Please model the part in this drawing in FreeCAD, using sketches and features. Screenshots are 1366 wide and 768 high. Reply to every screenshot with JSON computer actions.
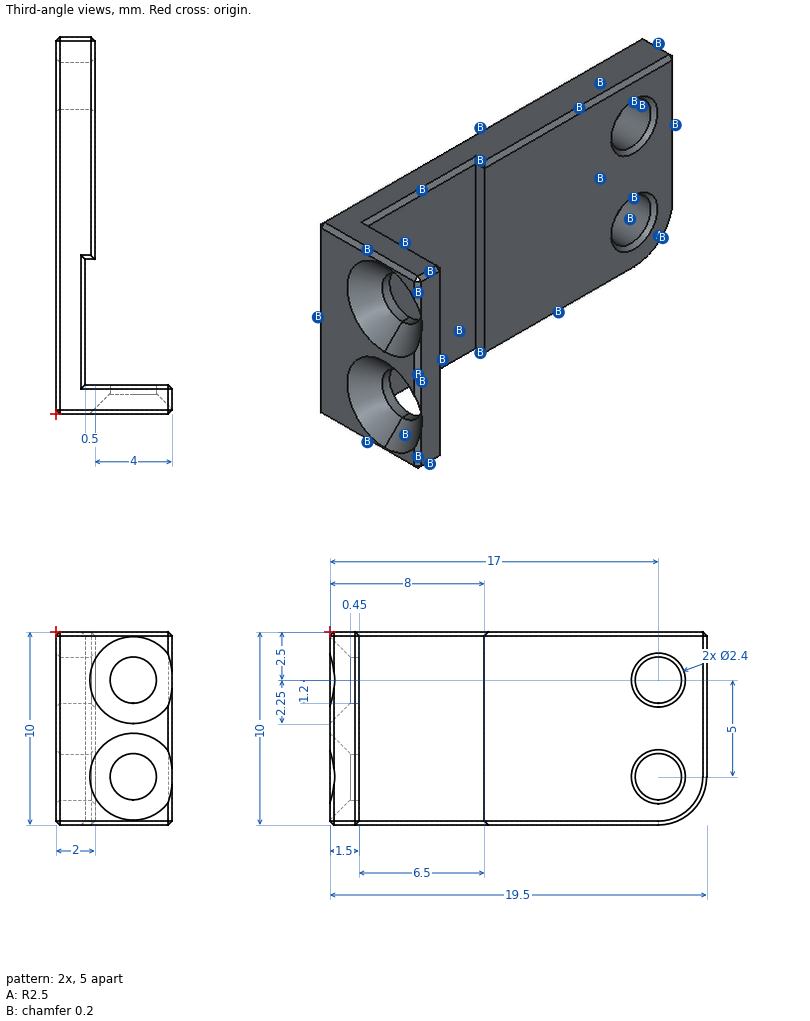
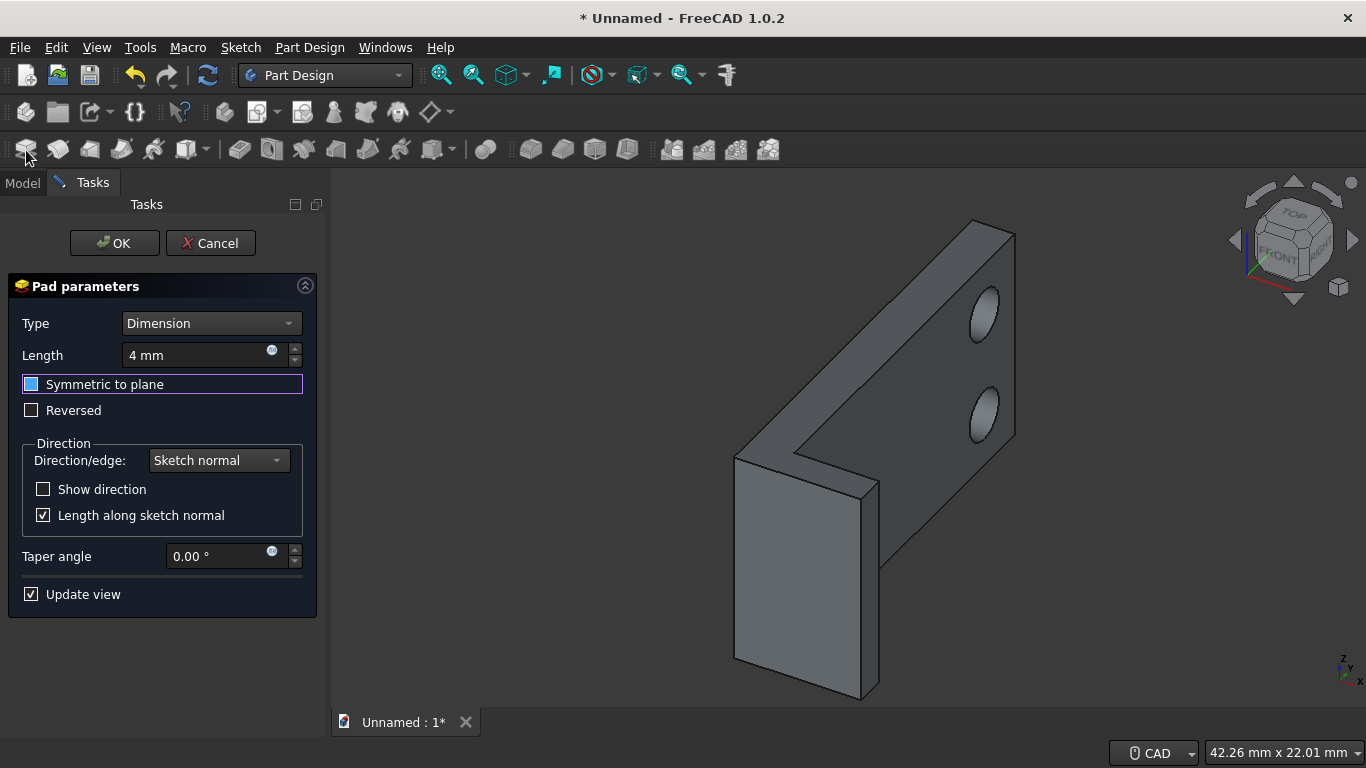
{"action": "left_click", "coordinate": [115, 243]}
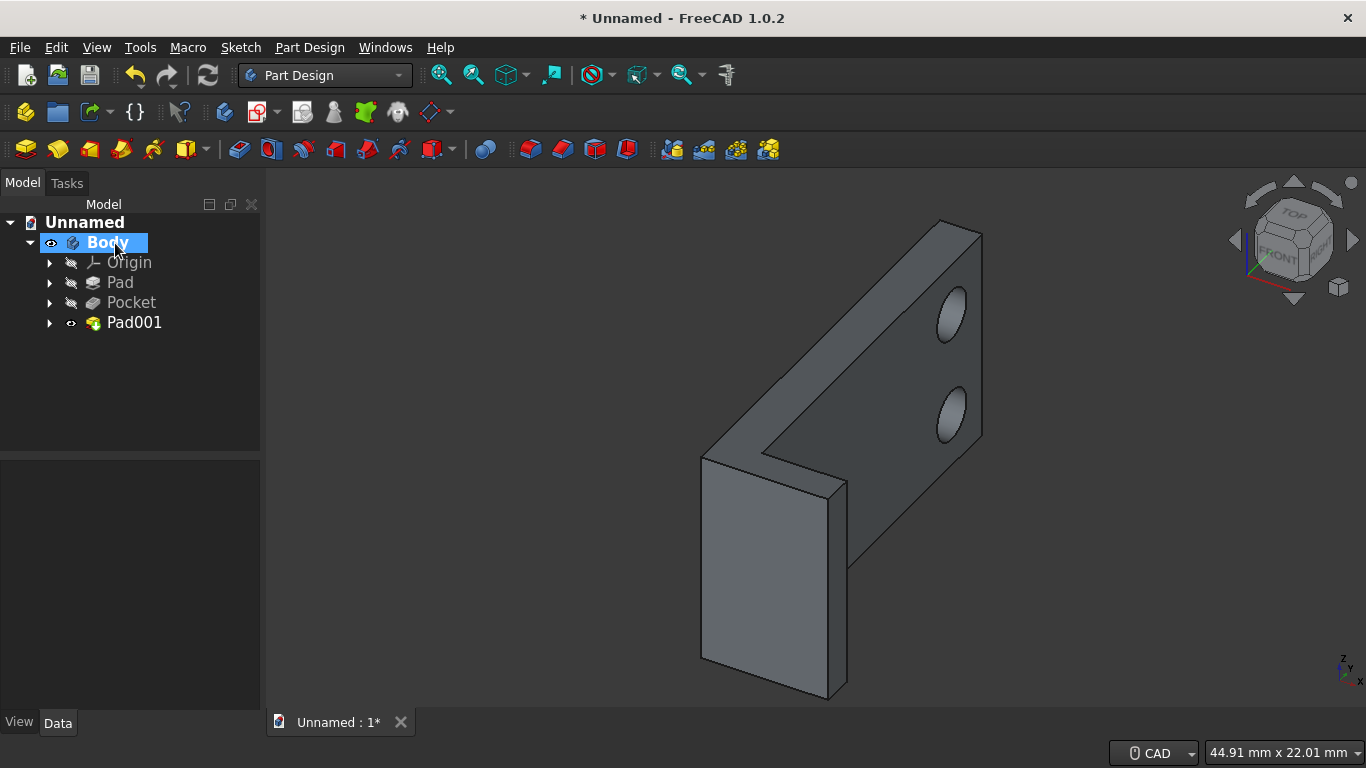
{"action": "left_click", "coordinate": [872, 443]}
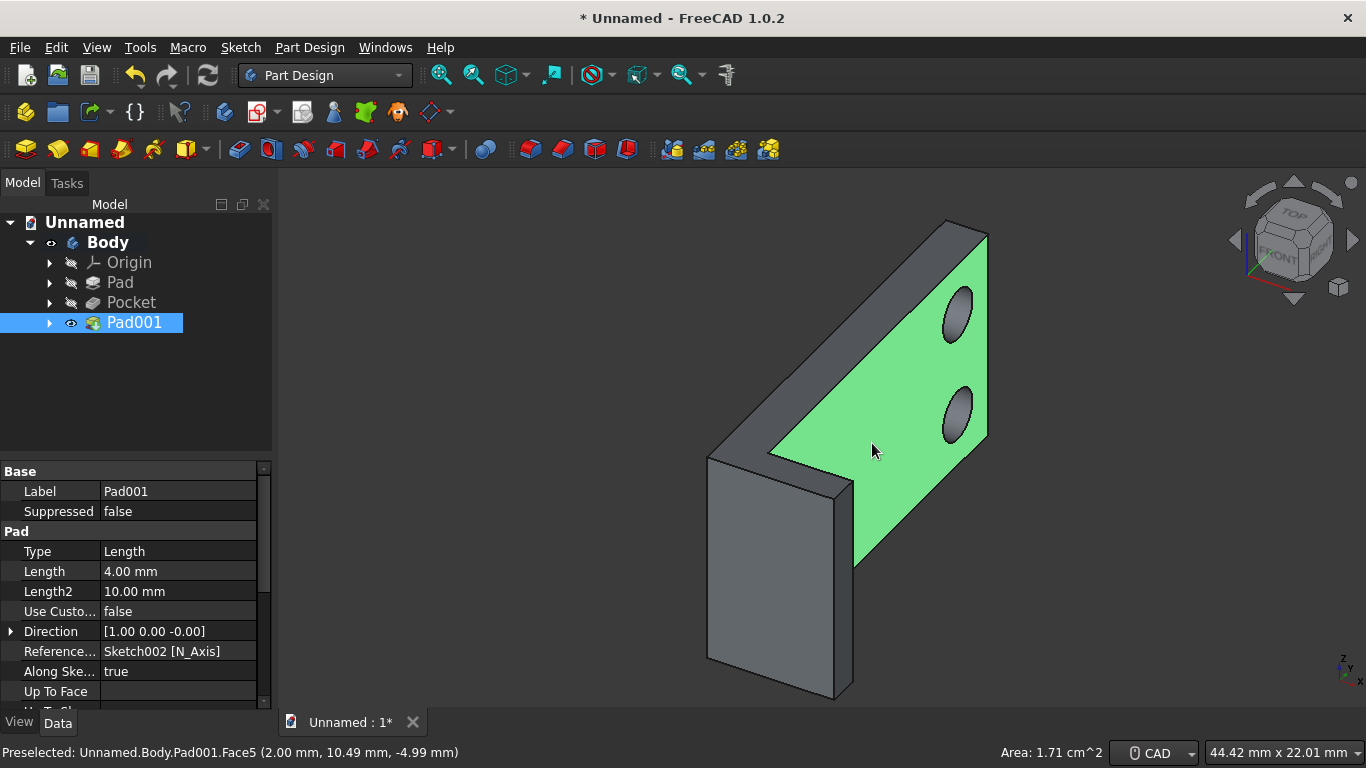
{"action": "left_click", "coordinate": [258, 112]}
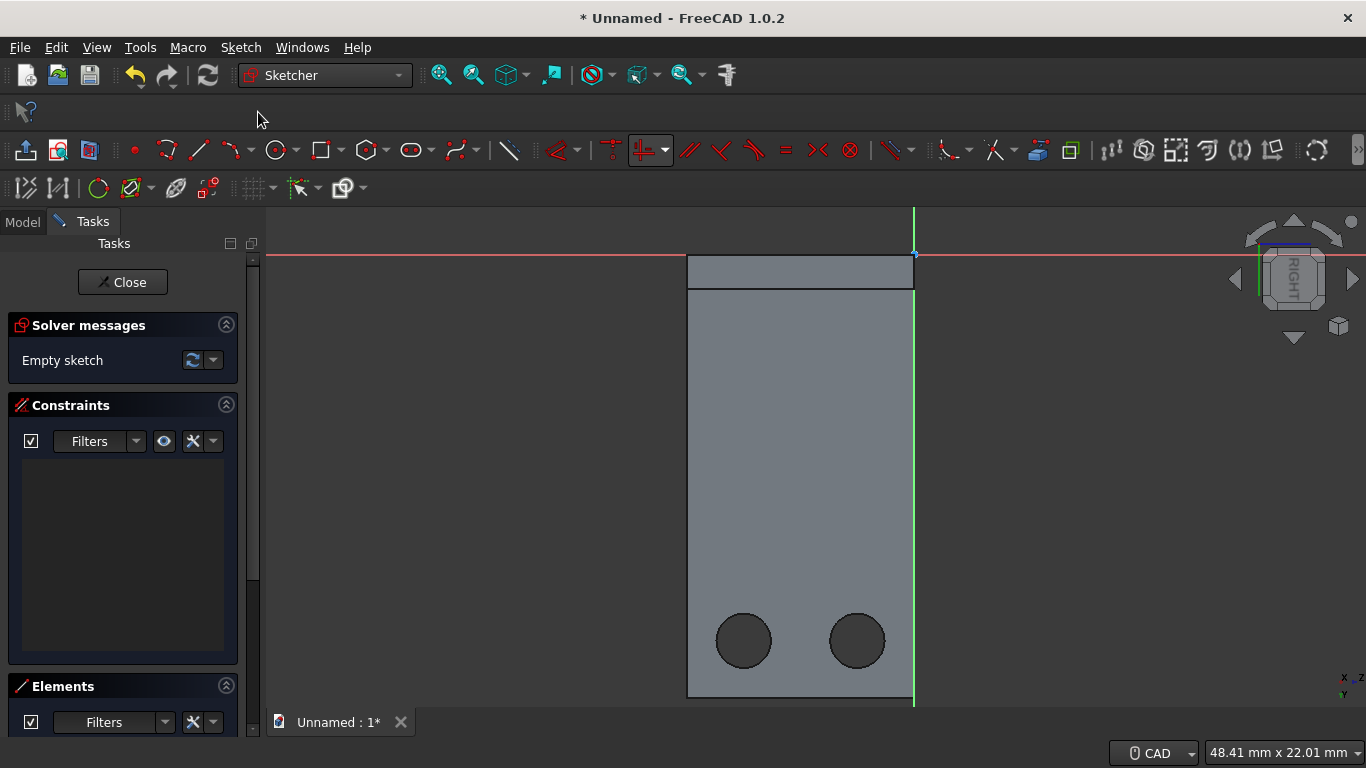
{"action": "scroll", "coordinate": [865, 235], "scroll_direction": "up", "scroll_amount": 3}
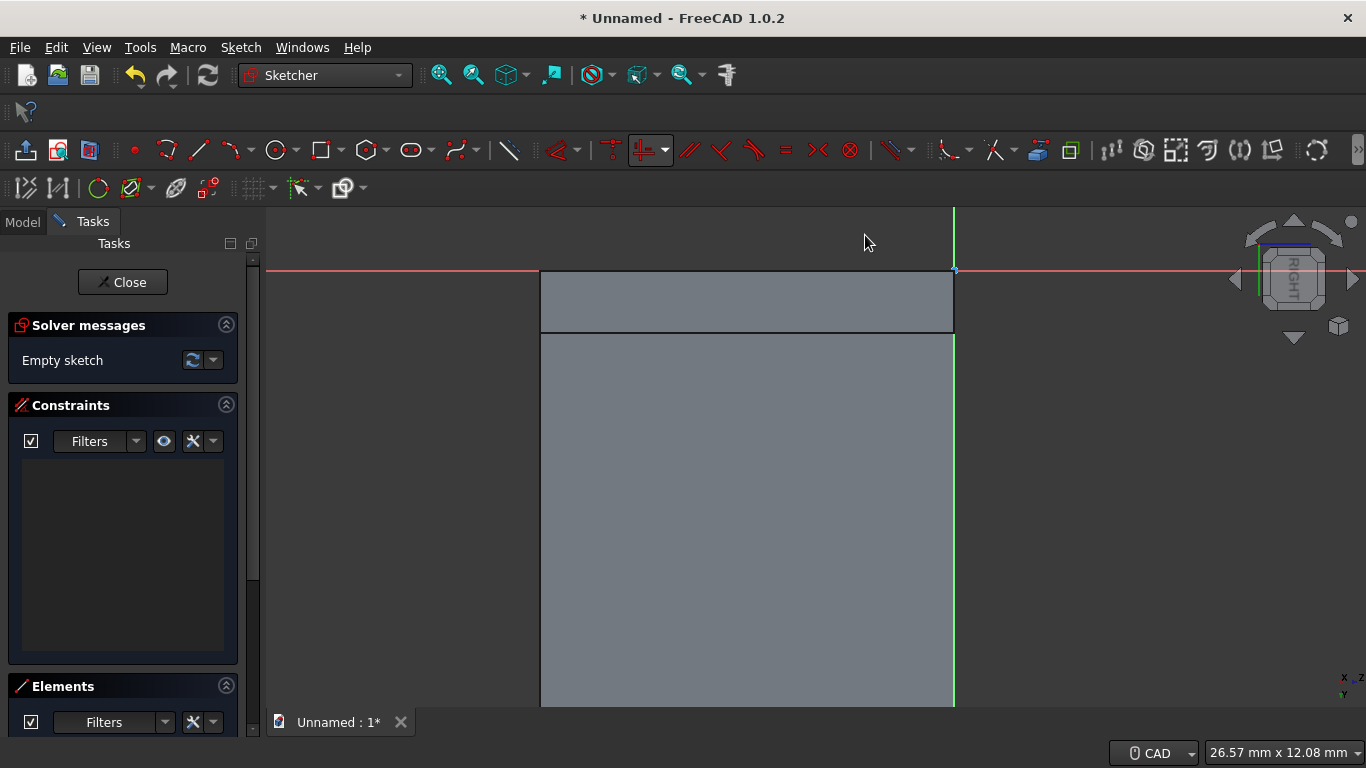
{"action": "left_click", "coordinate": [322, 150]}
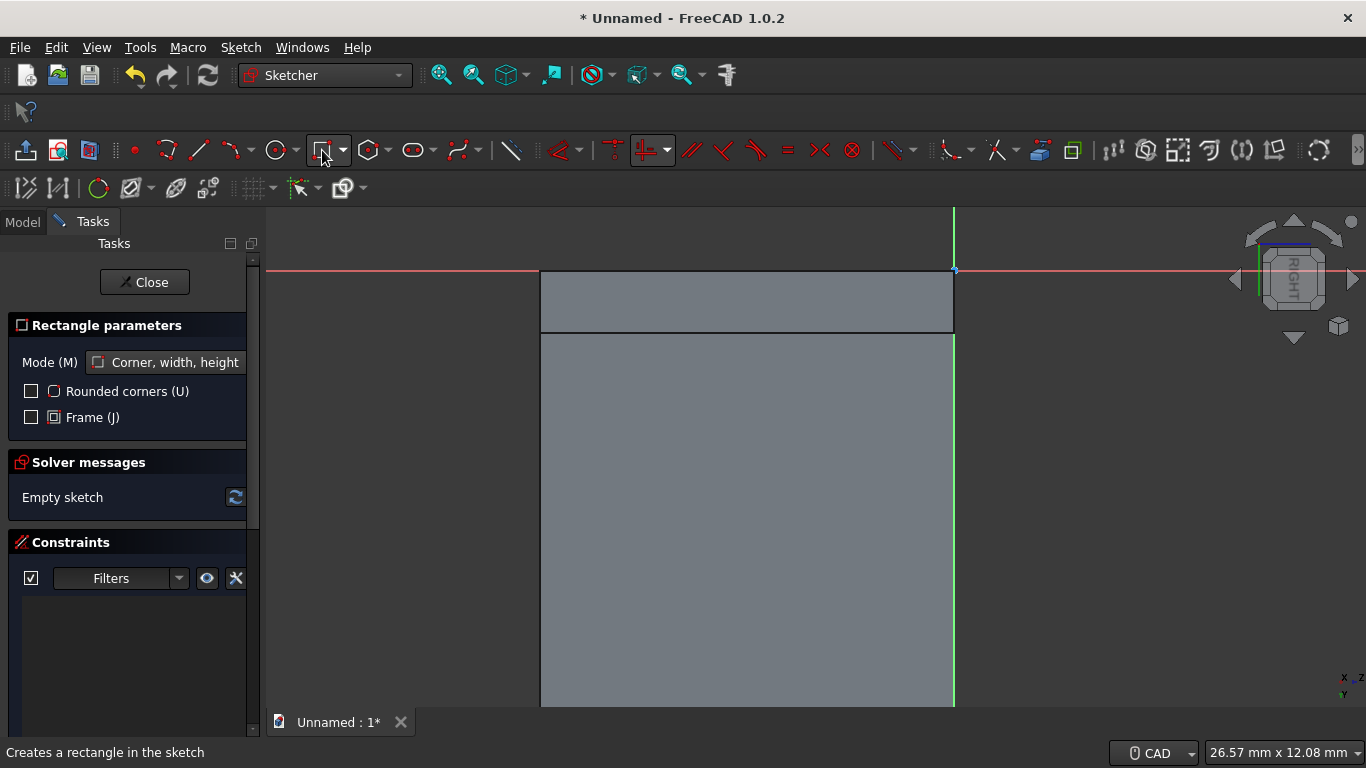
{"action": "left_click", "coordinate": [540, 333]}
{"action": "left_click", "coordinate": [954, 602]}
{"action": "key", "text": "Escape"}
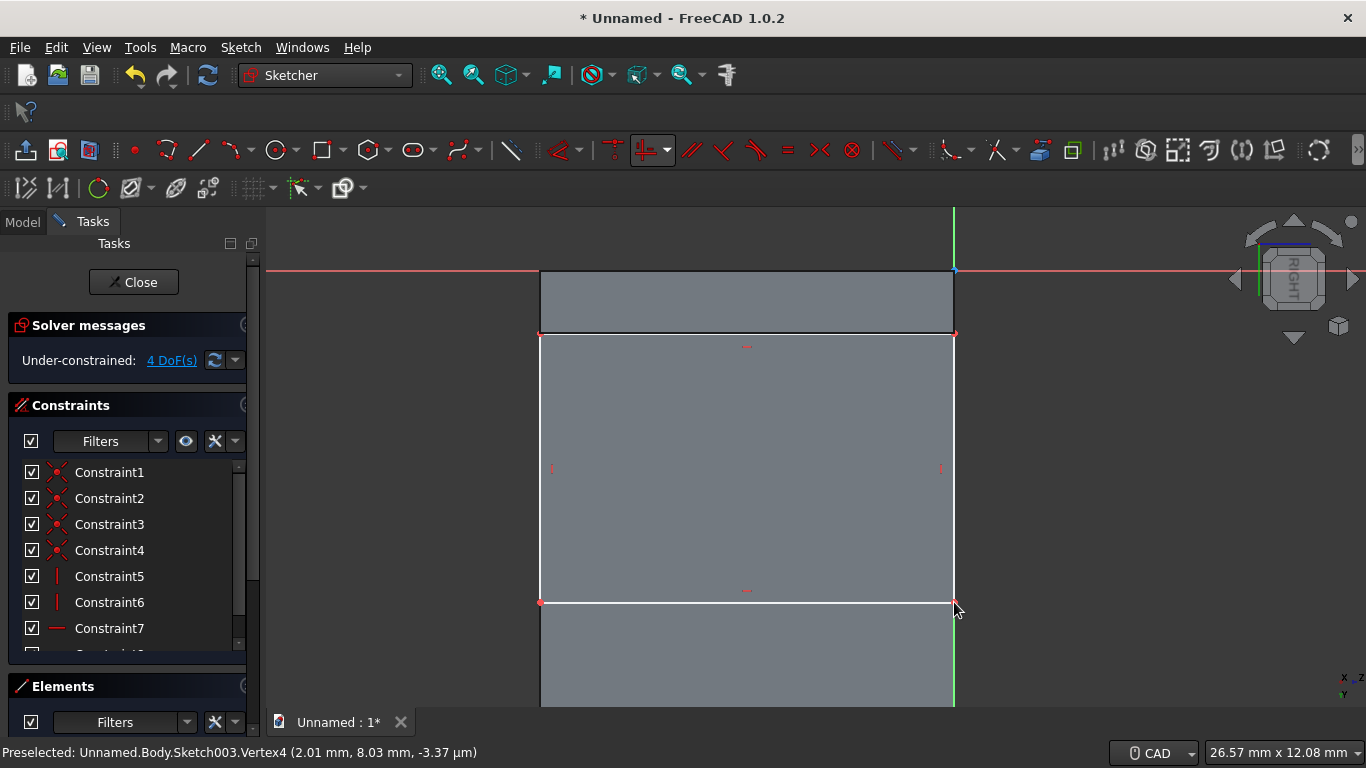
{"action": "left_click", "coordinate": [954, 603]}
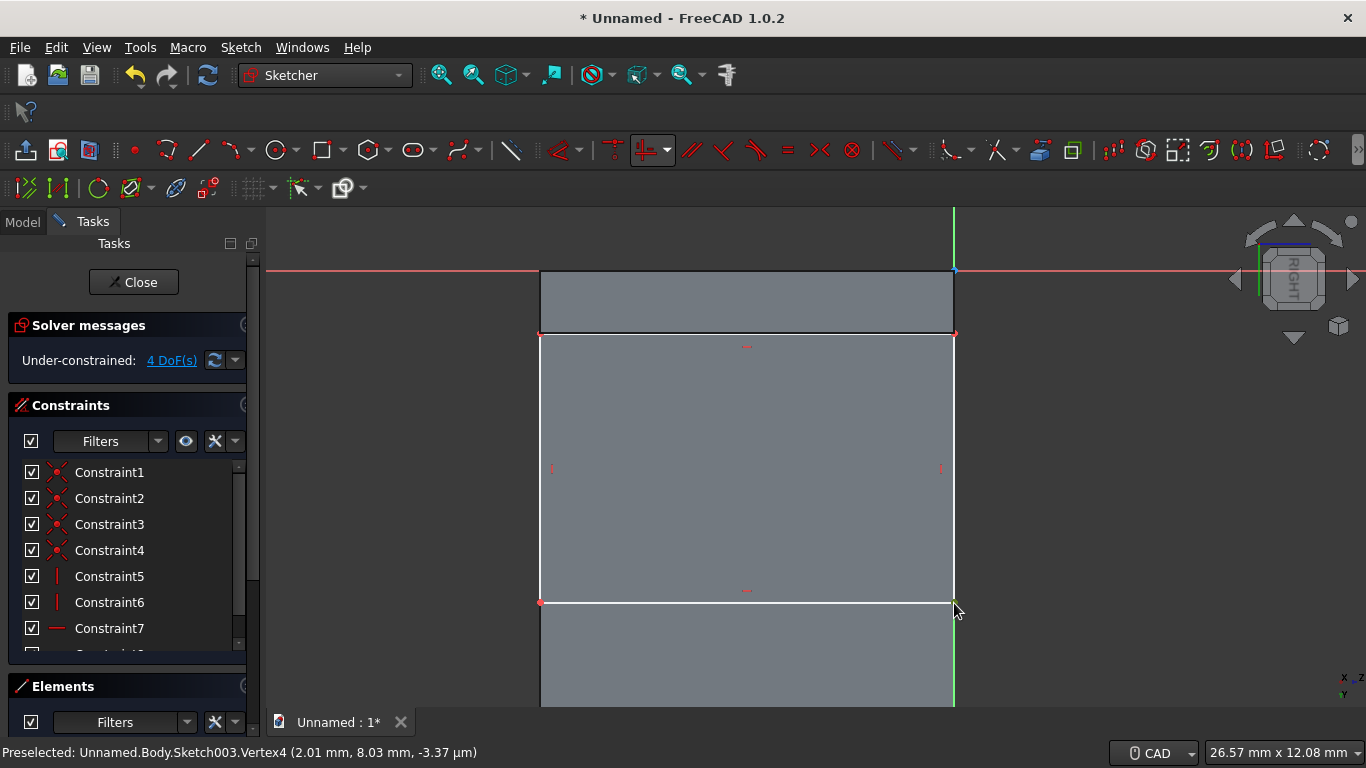
{"action": "left_click", "coordinate": [954, 647]}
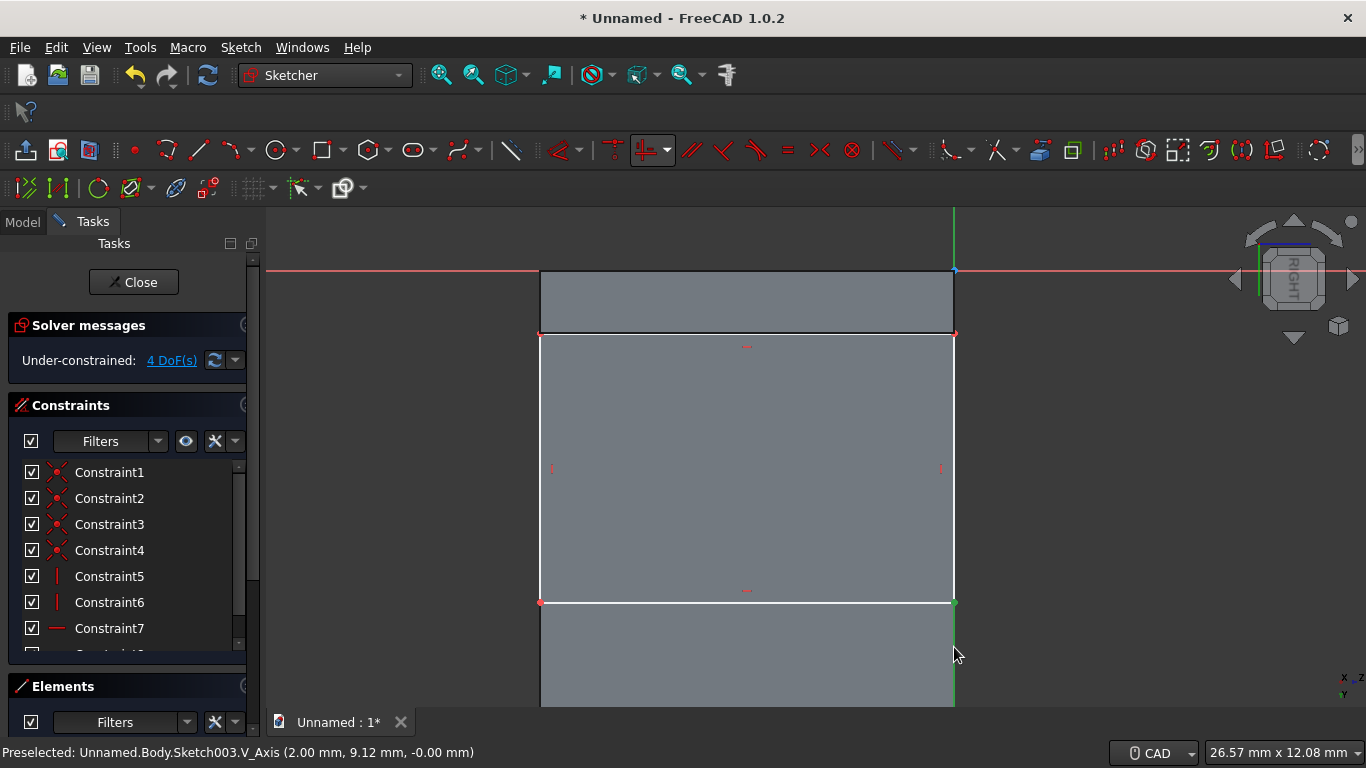
{"action": "left_click", "coordinate": [614, 150]}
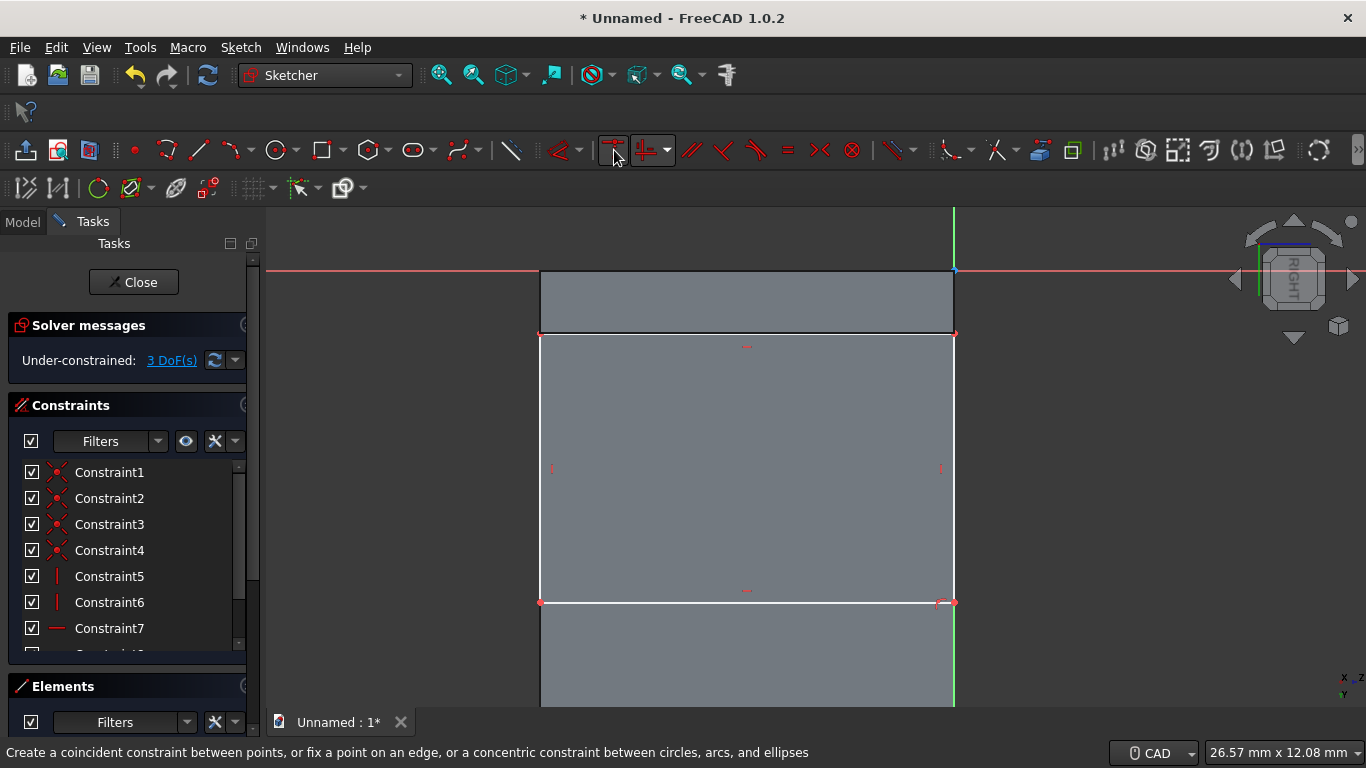
{"action": "left_click", "coordinate": [558, 150]}